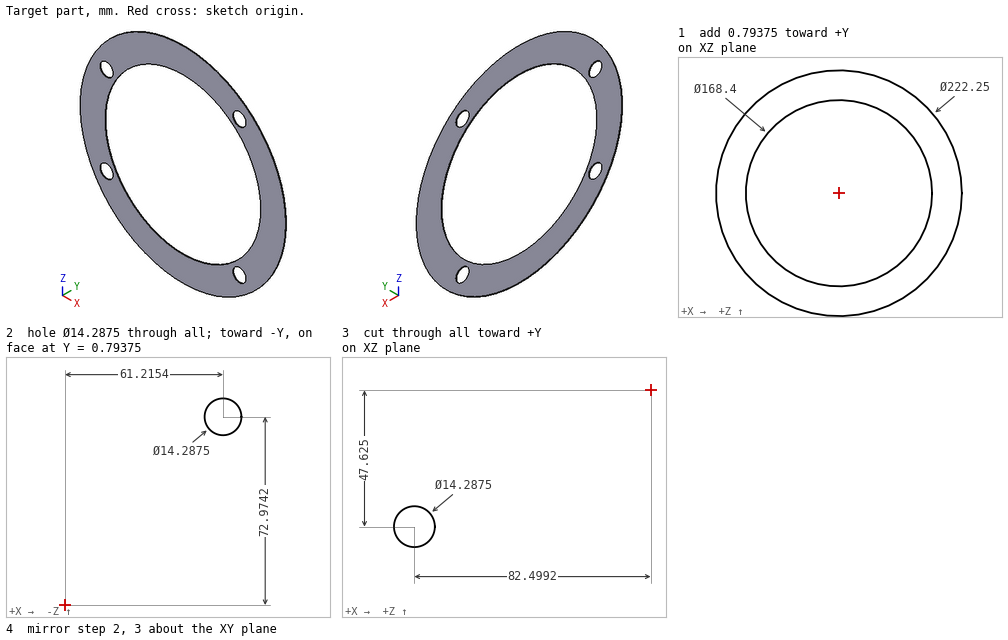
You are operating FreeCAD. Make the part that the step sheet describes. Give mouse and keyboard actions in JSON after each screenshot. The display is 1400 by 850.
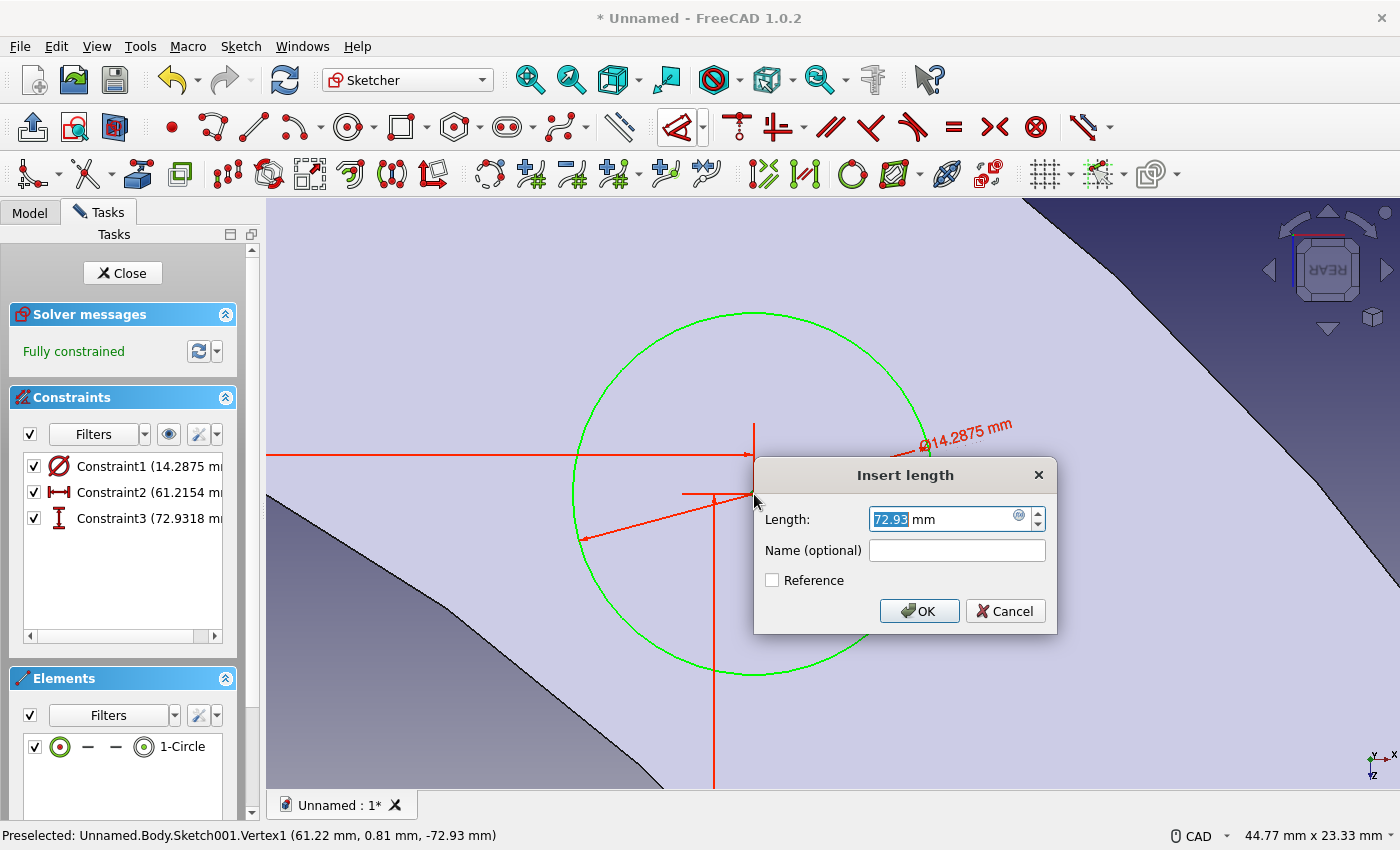
{"action": "type", "text": "72.9742"}
{"action": "key", "text": "Return"}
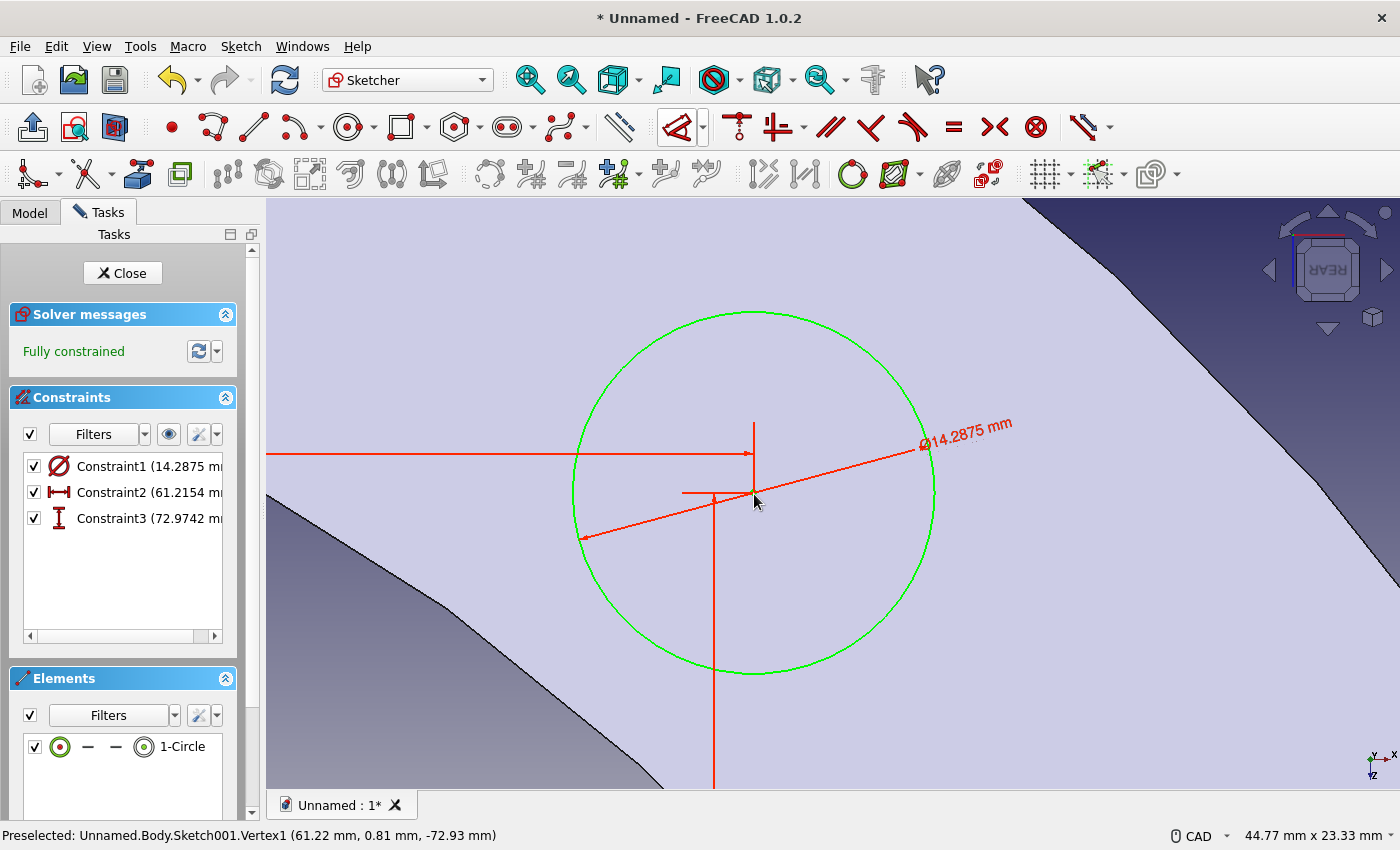
{"action": "left_click", "coordinate": [123, 273]}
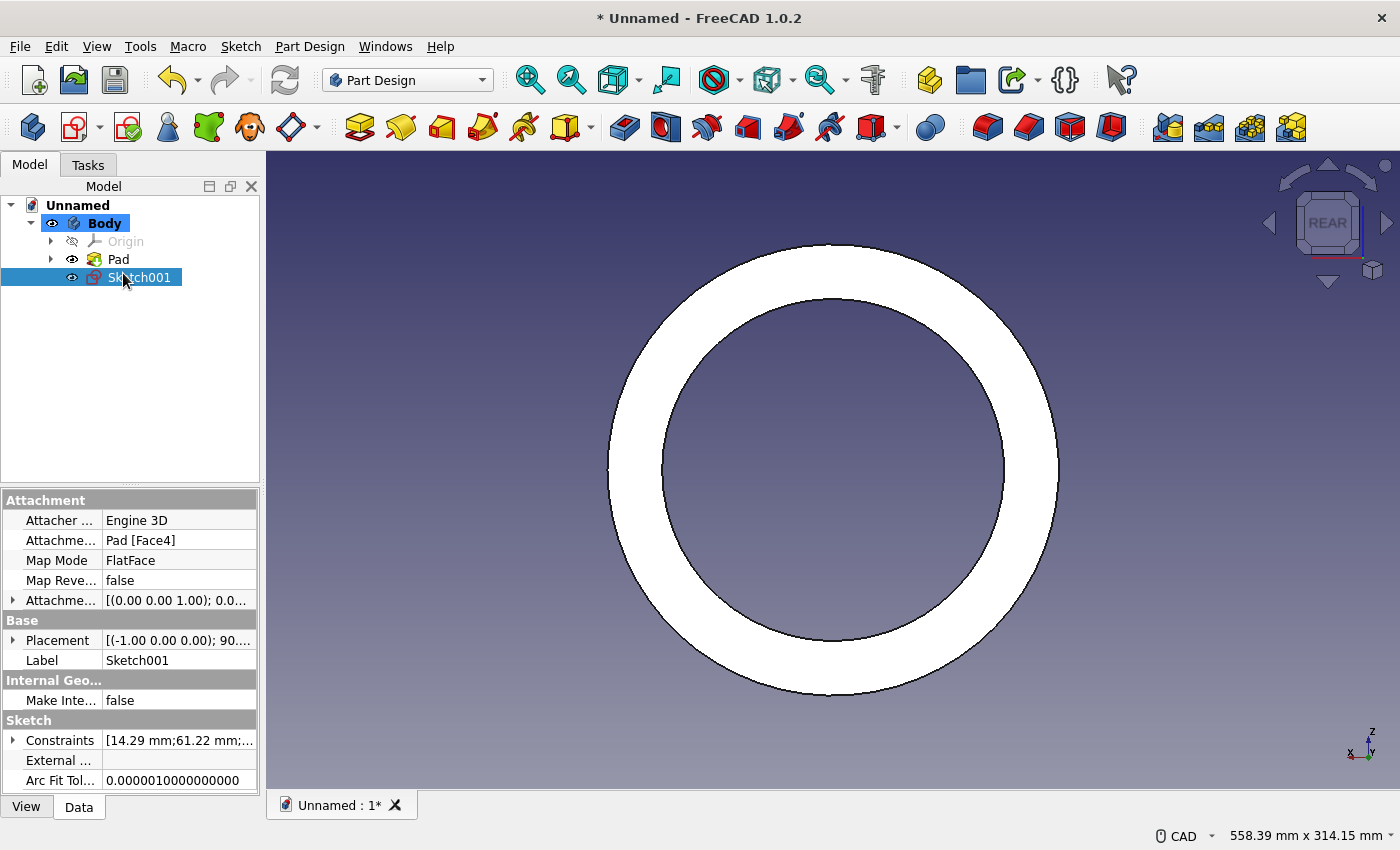
{"action": "left_click", "coordinate": [666, 128]}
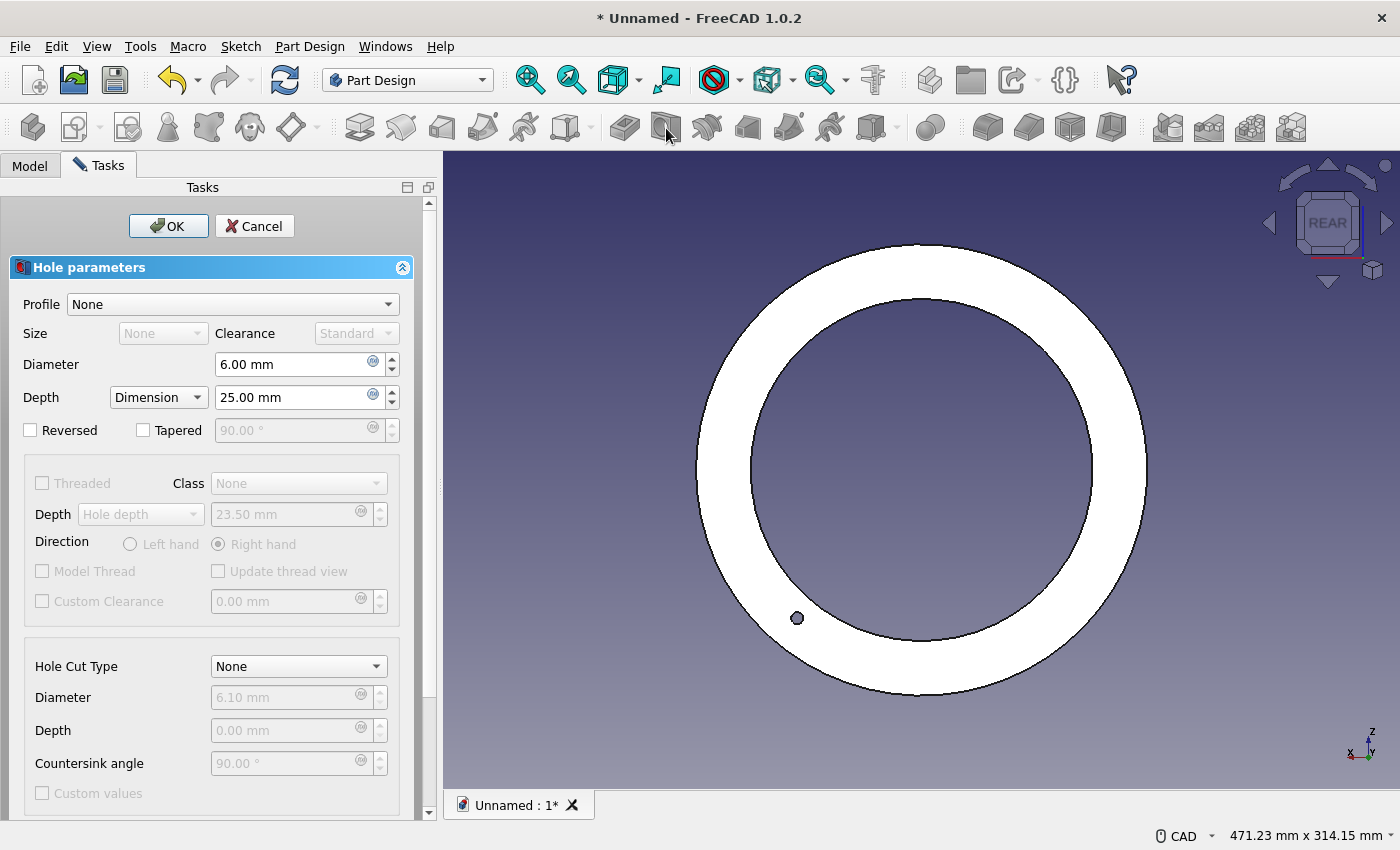
{"action": "triple_click", "coordinate": [300, 364]}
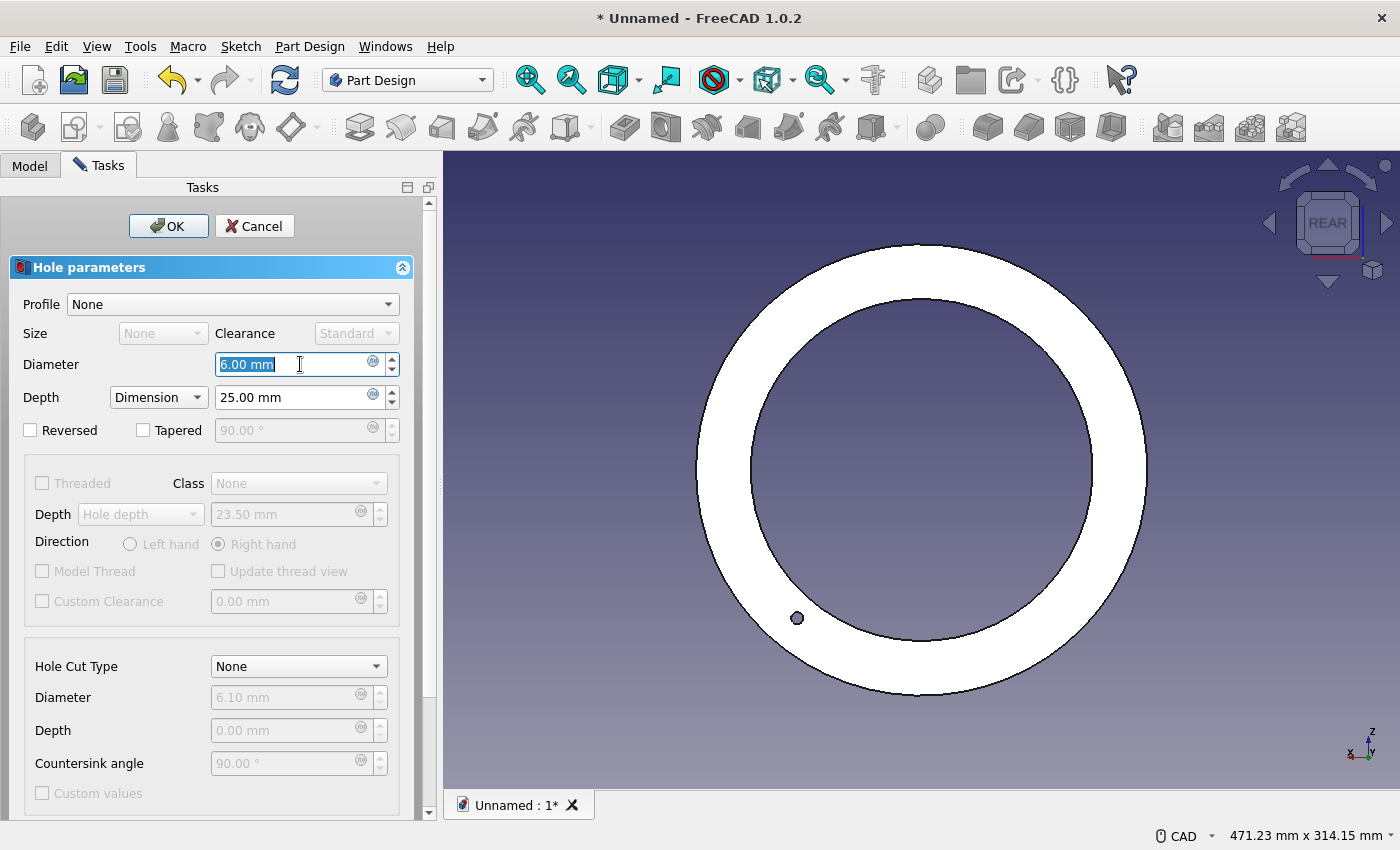
{"action": "type", "text": "14.2875"}
{"action": "key", "text": "Tab"}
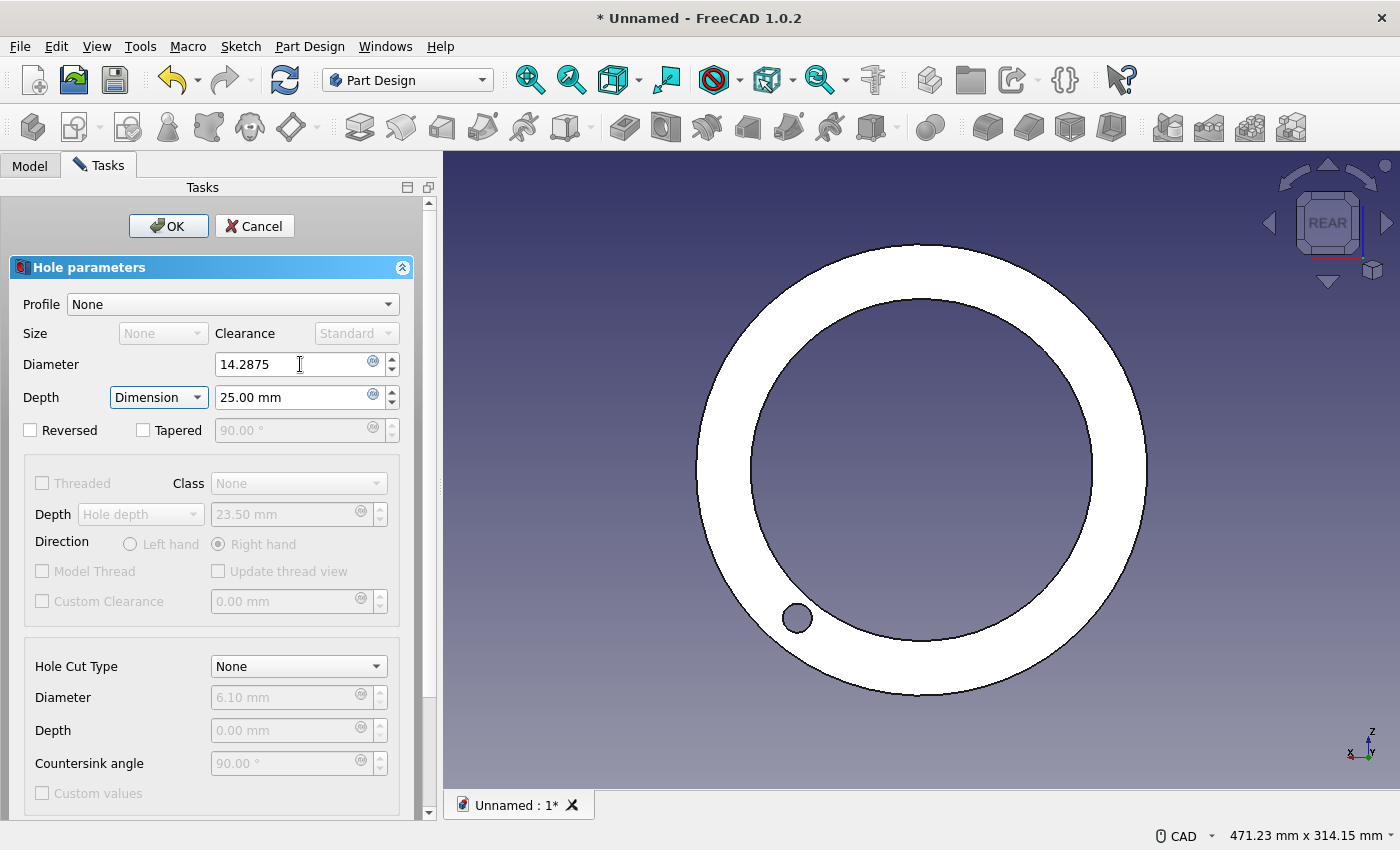
{"action": "left_click", "coordinate": [160, 398]}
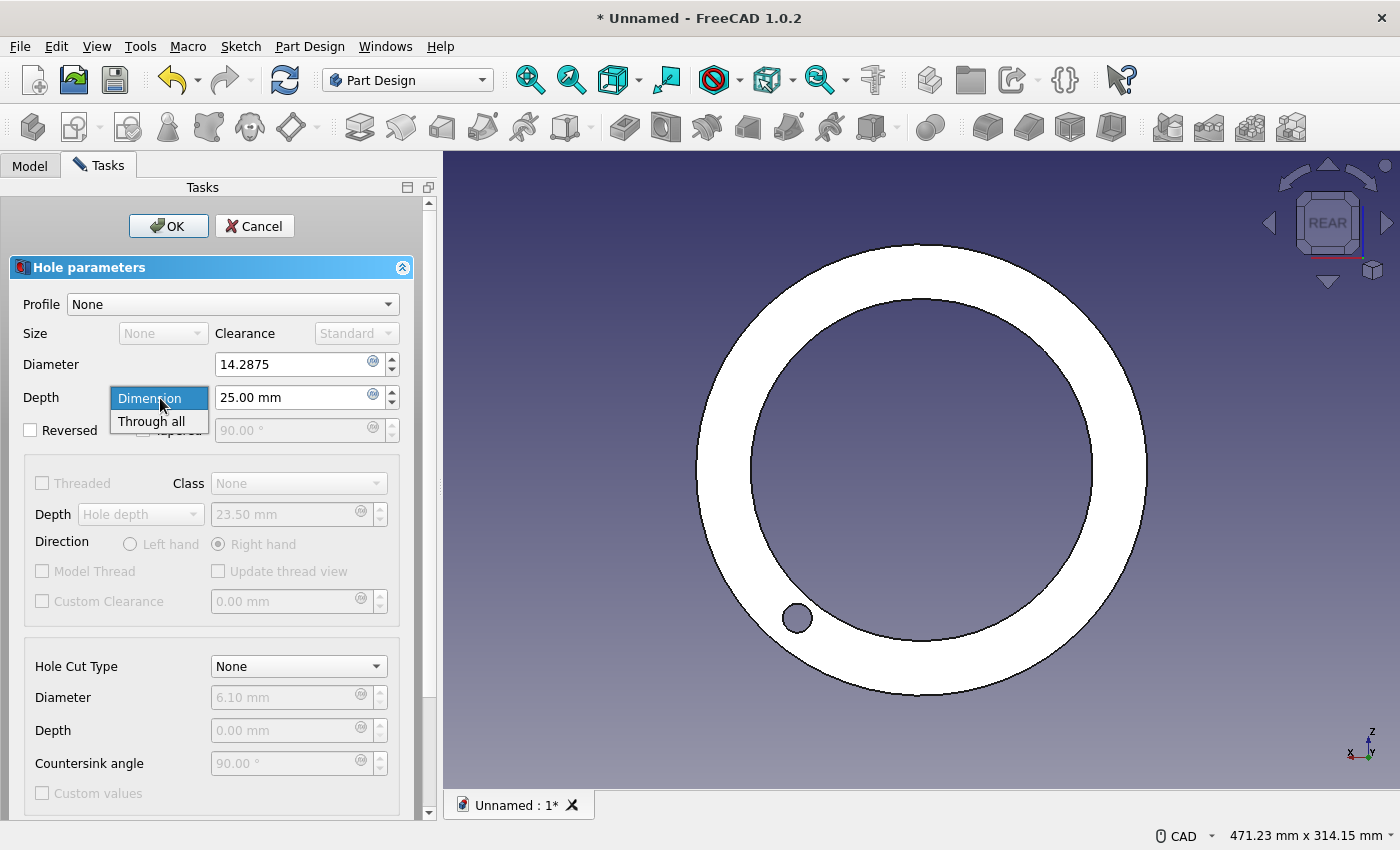
{"action": "left_click", "coordinate": [158, 422]}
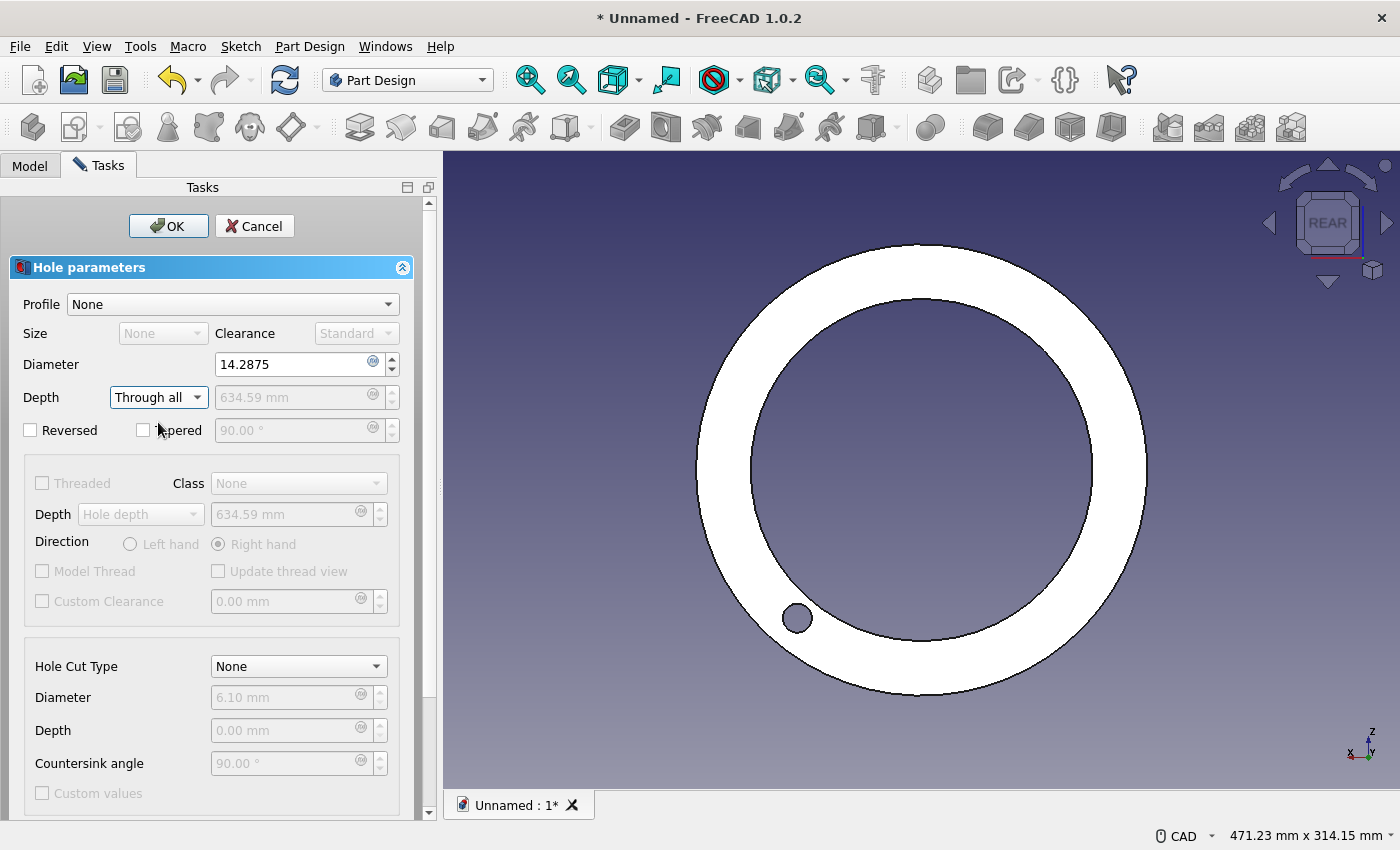
{"action": "left_click", "coordinate": [169, 226]}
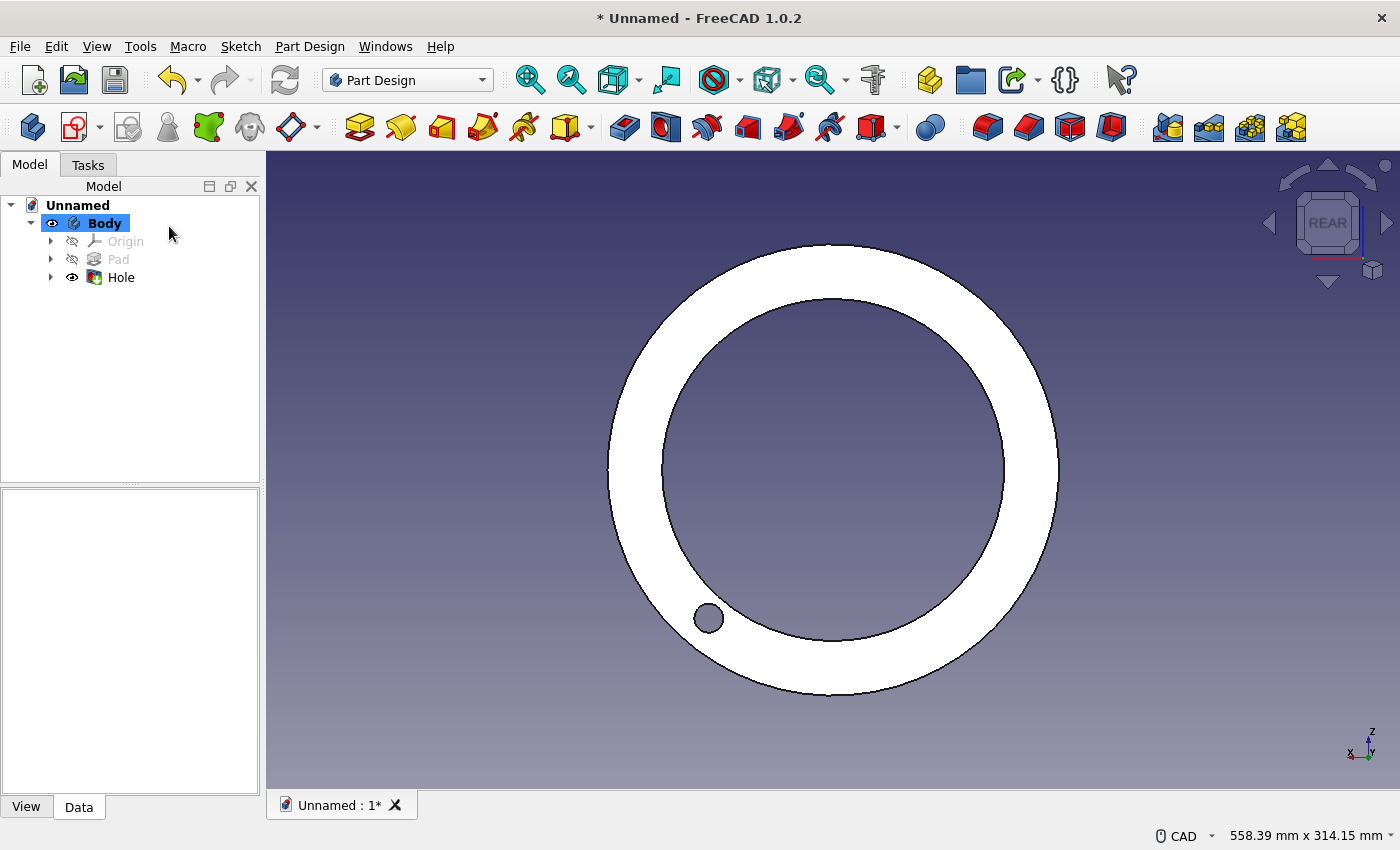
{"action": "left_click", "coordinate": [74, 128]}